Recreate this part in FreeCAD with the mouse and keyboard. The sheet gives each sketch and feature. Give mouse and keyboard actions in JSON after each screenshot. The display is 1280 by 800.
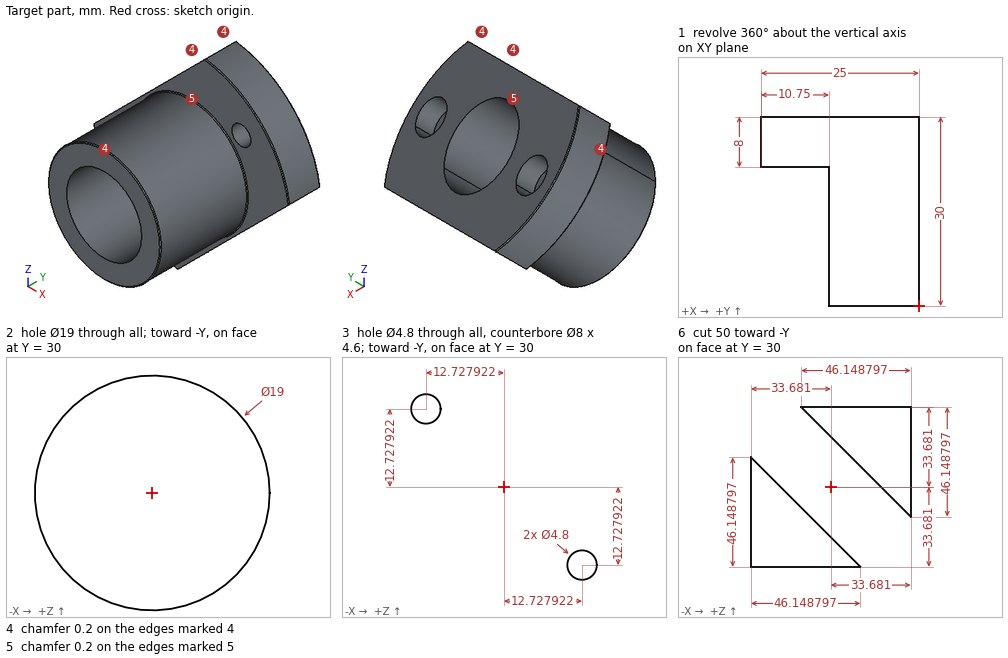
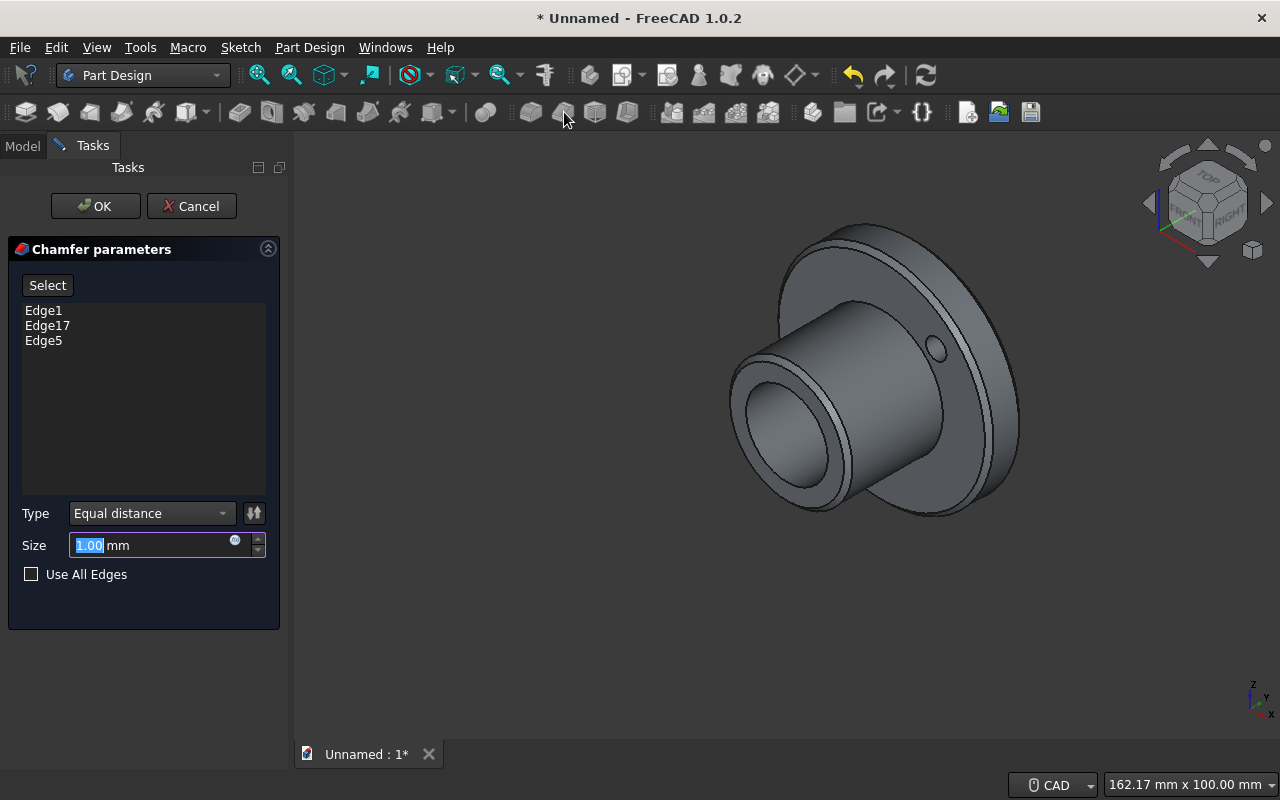
{"action": "type", "text": "0.2"}
{"action": "key", "text": "Tab"}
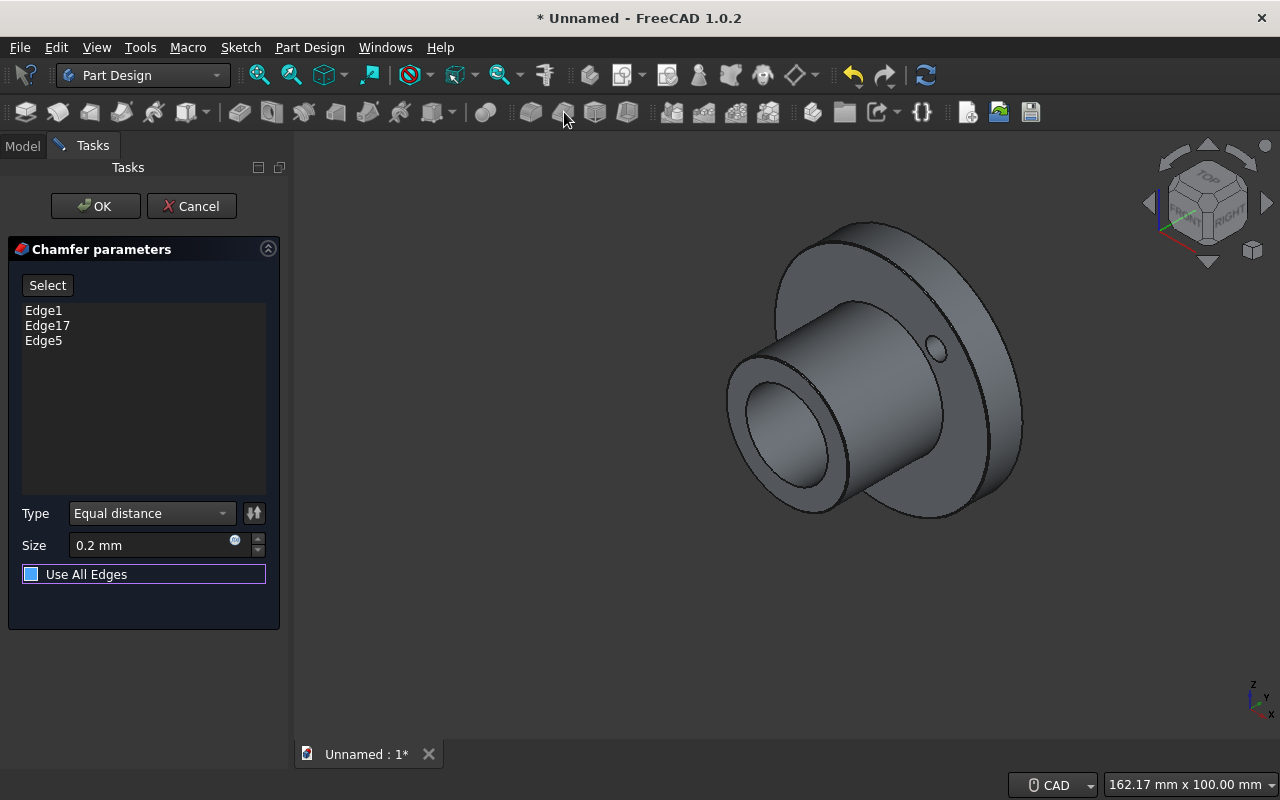
{"action": "left_click", "coordinate": [96, 206]}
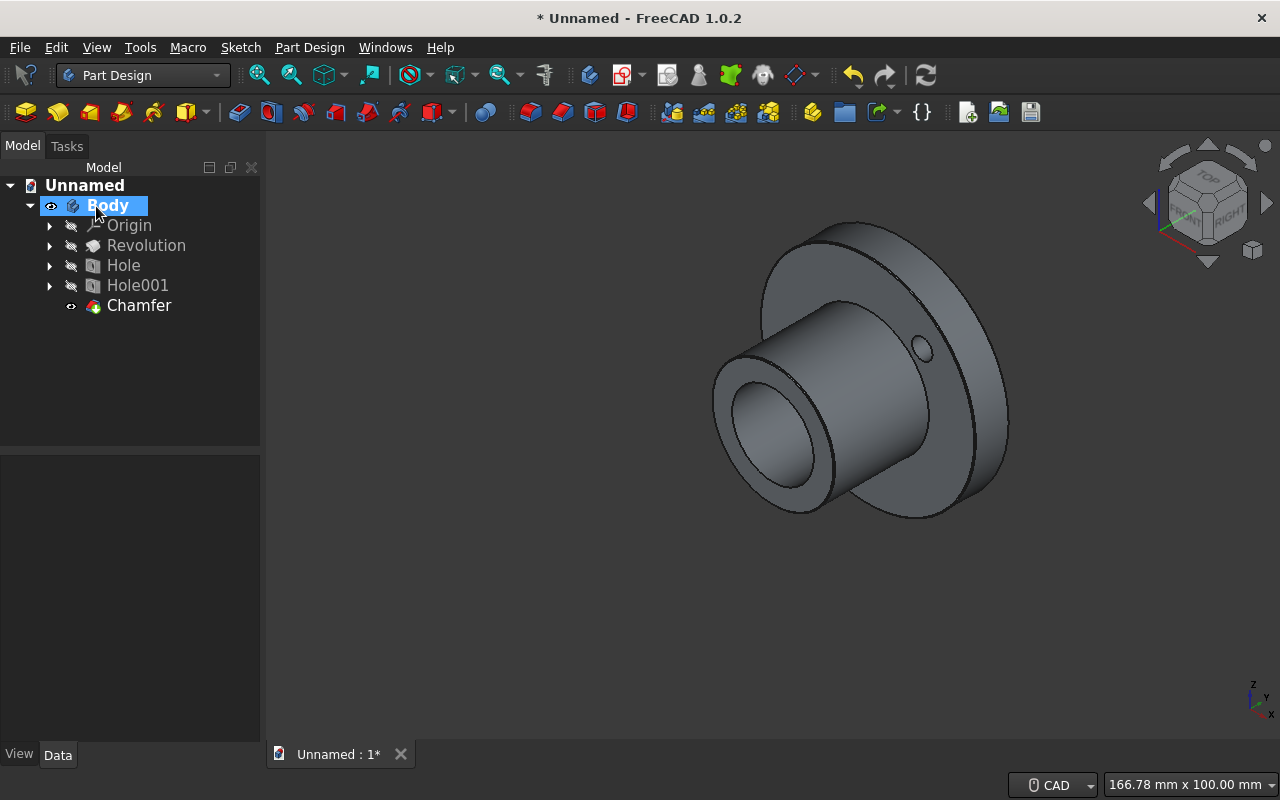
{"action": "key", "text": "2"}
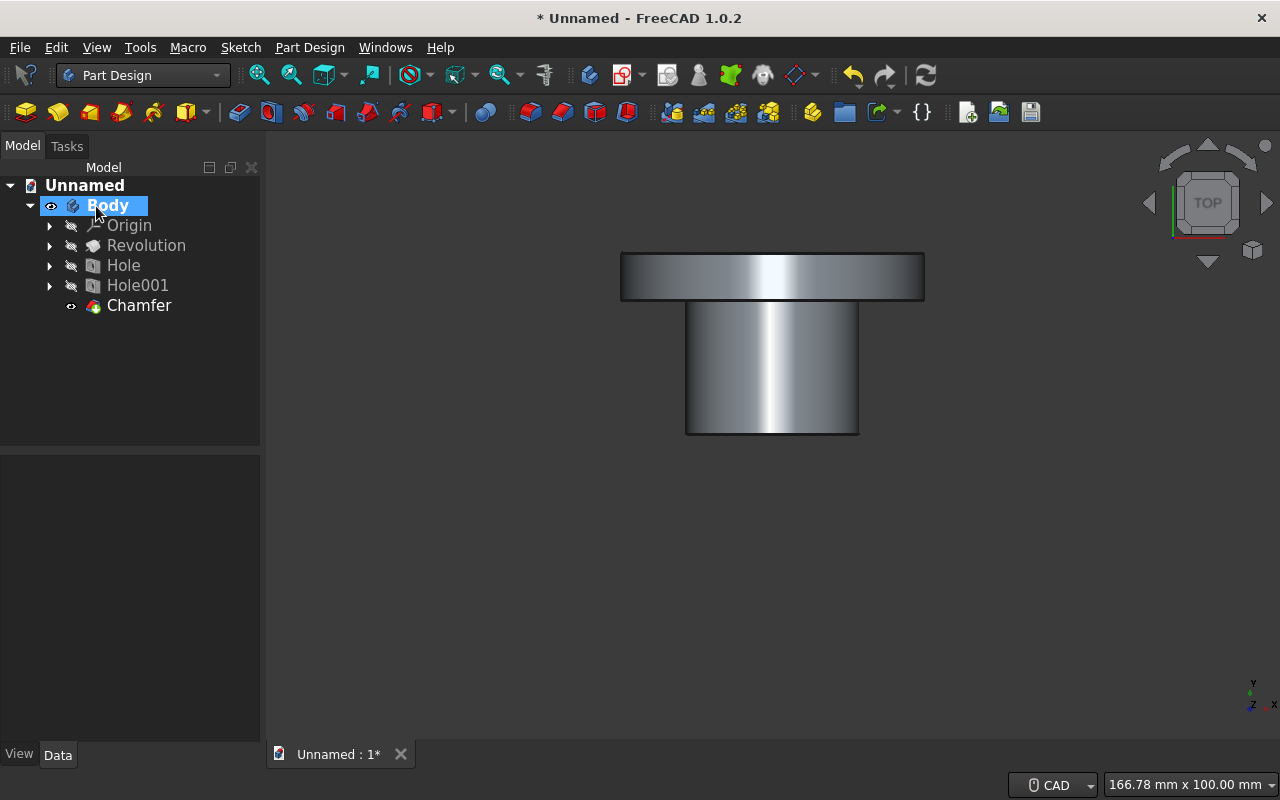
{"action": "left_click", "coordinate": [260, 76]}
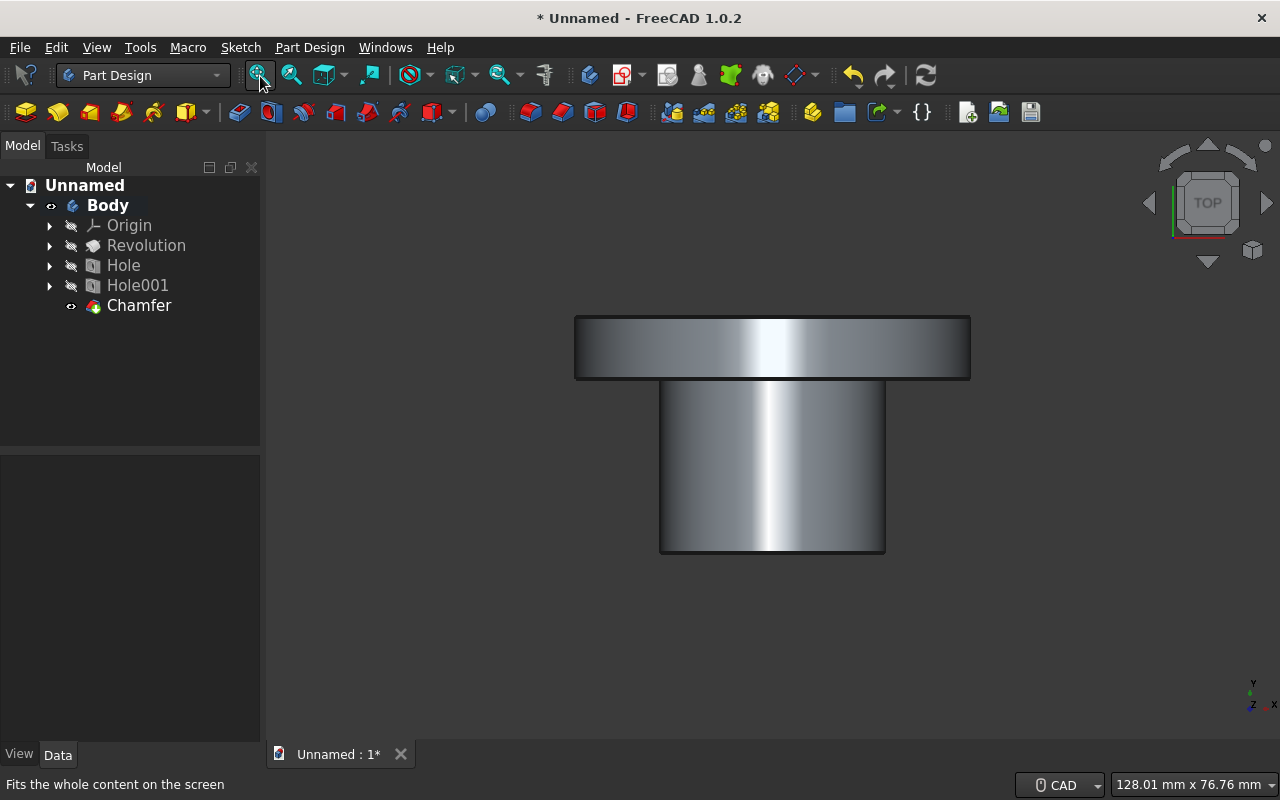
{"action": "key", "text": "0"}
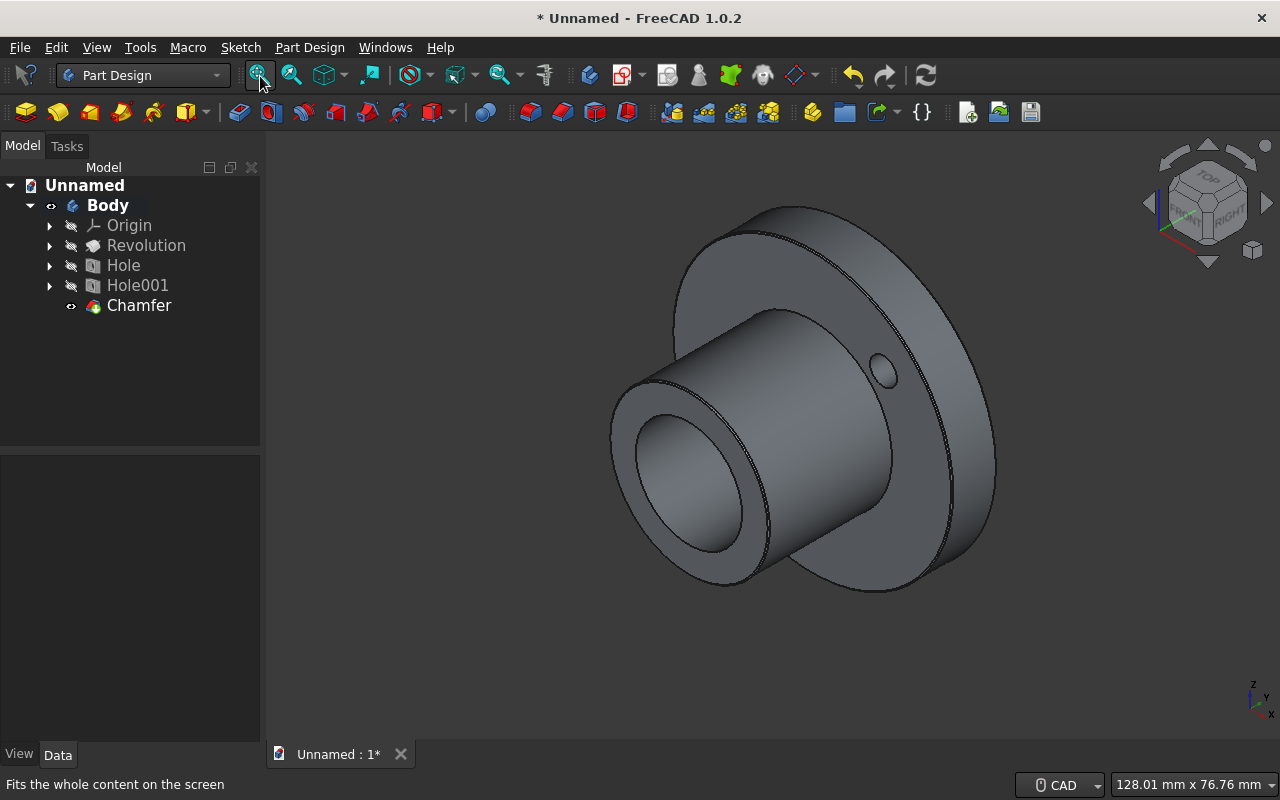
{"action": "key", "text": "1"}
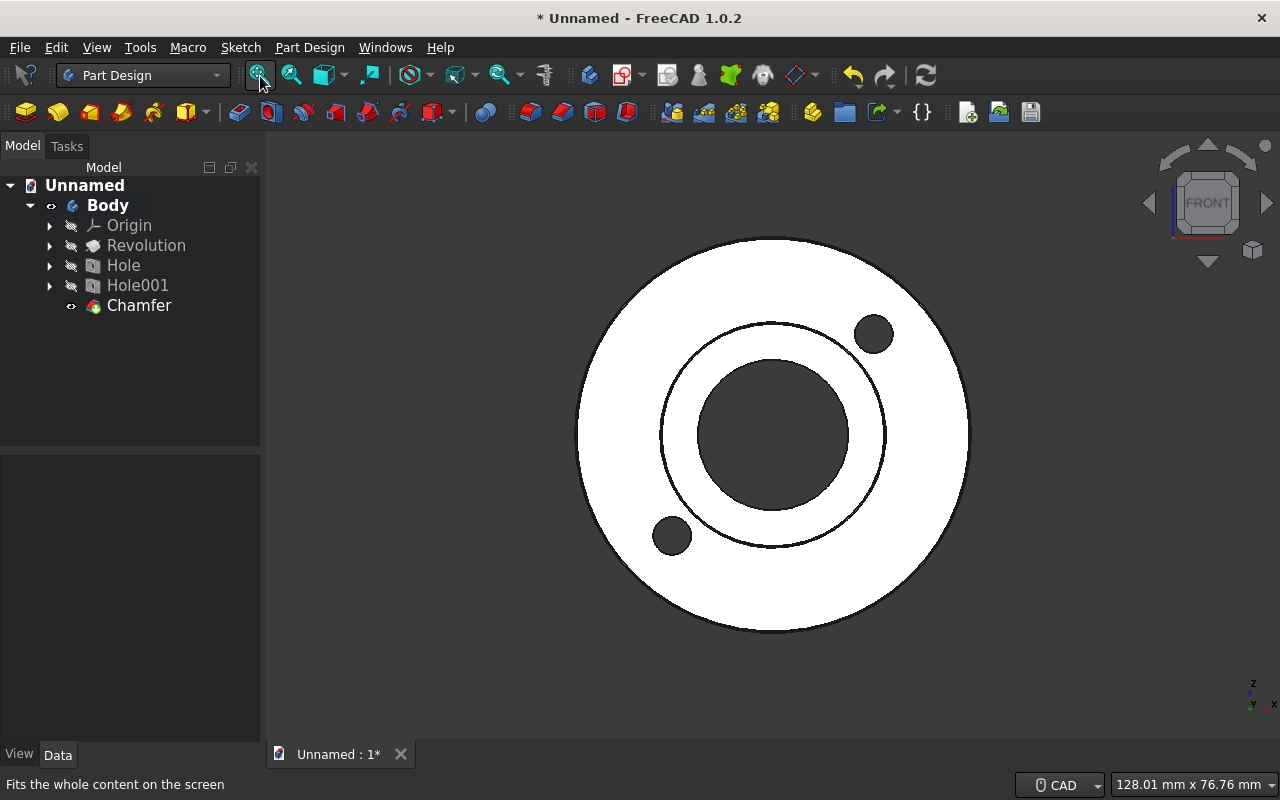
{"action": "key", "text": "3"}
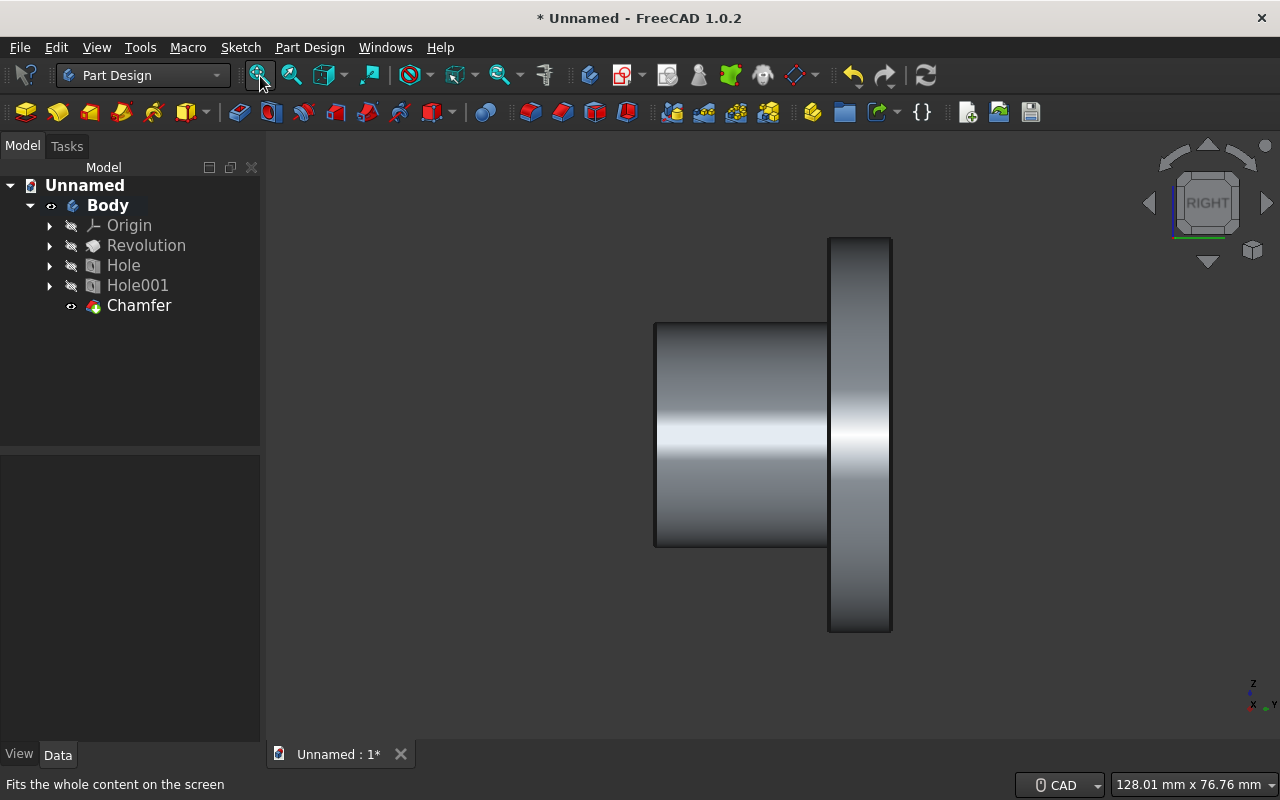
{"action": "key", "text": "5"}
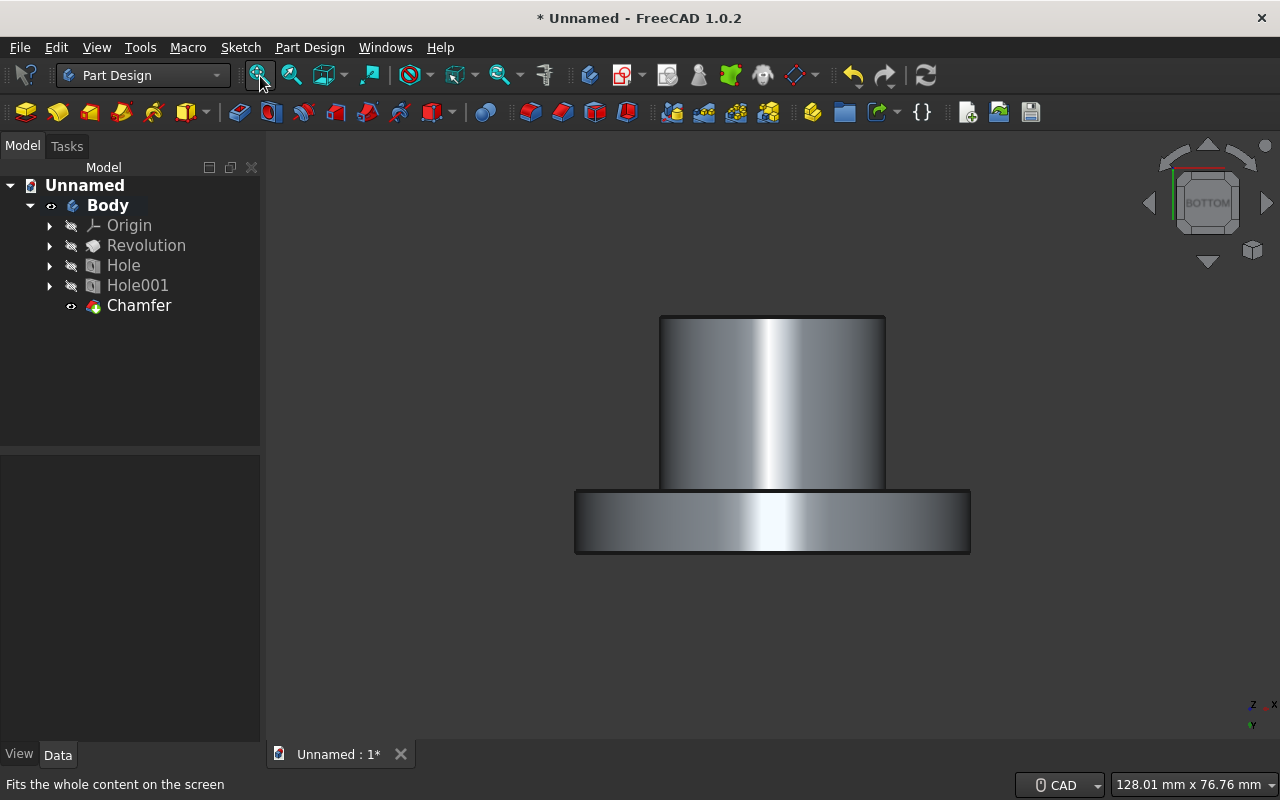
{"action": "left_click", "coordinate": [260, 76]}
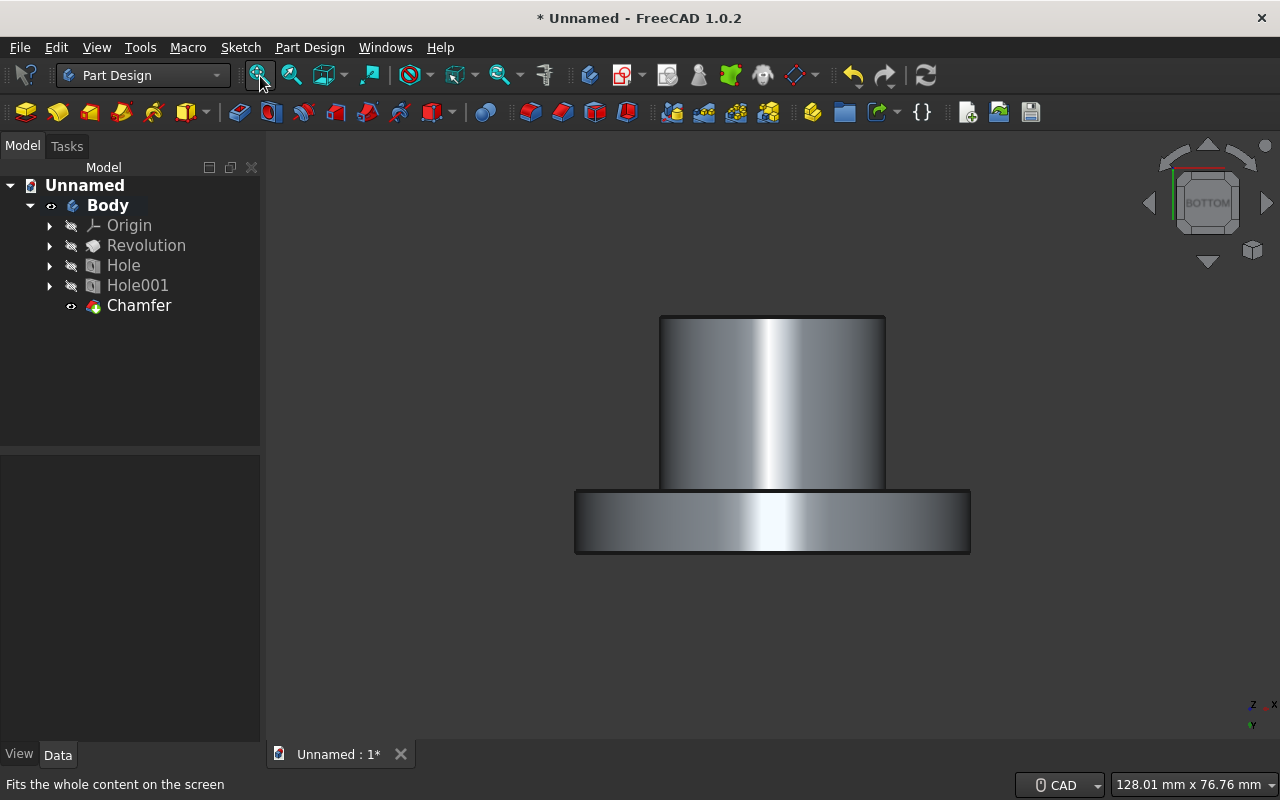
{"action": "key", "text": "4"}